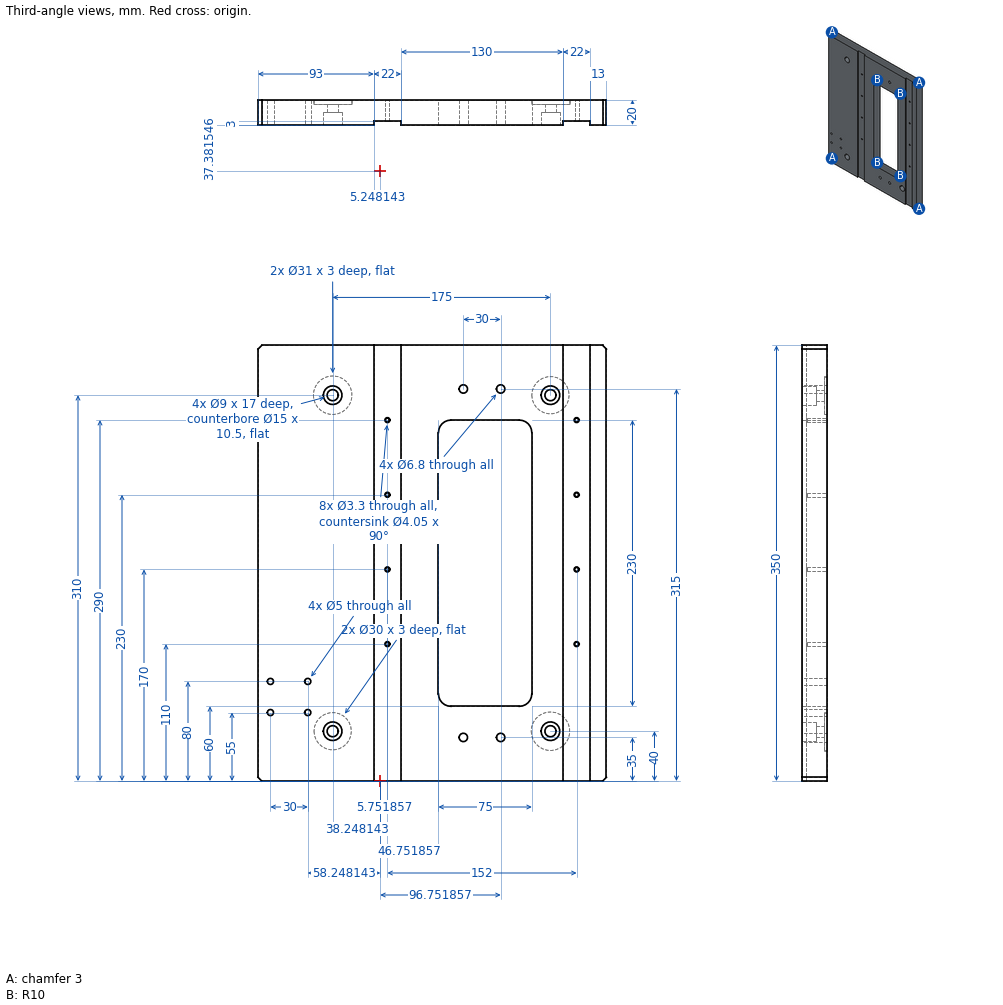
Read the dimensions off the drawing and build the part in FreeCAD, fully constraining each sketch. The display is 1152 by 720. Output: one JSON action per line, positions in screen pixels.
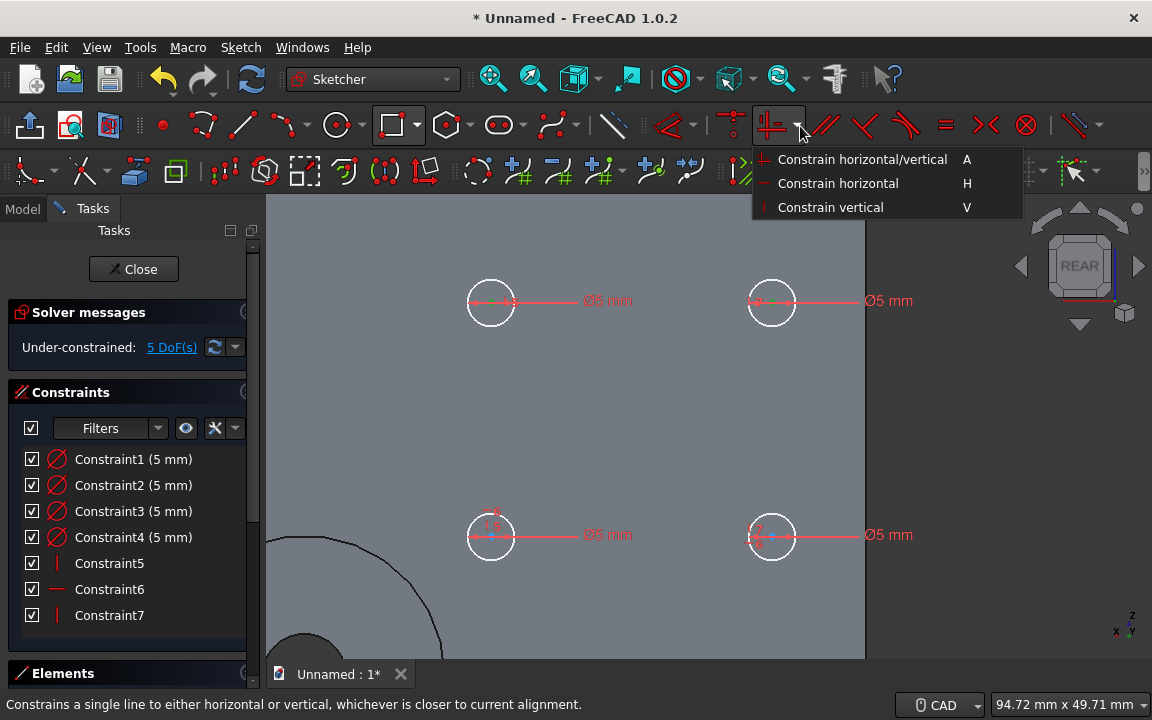
{"action": "left_click", "coordinate": [888, 183]}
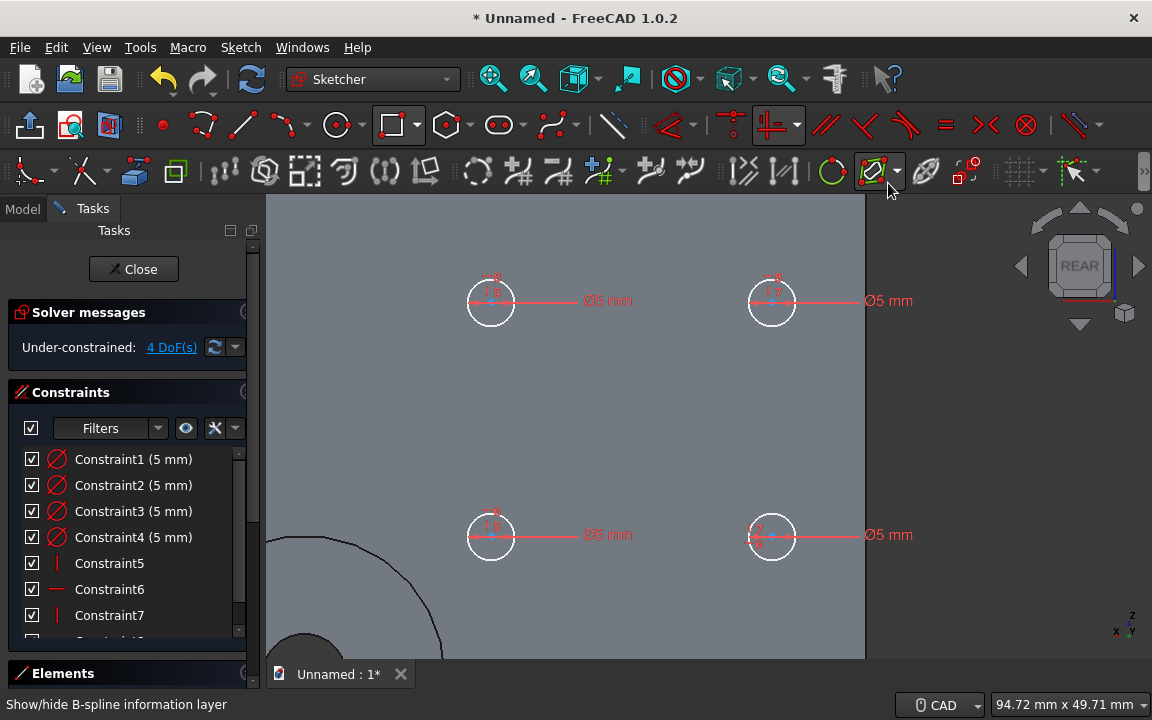
{"action": "left_click", "coordinate": [668, 126]}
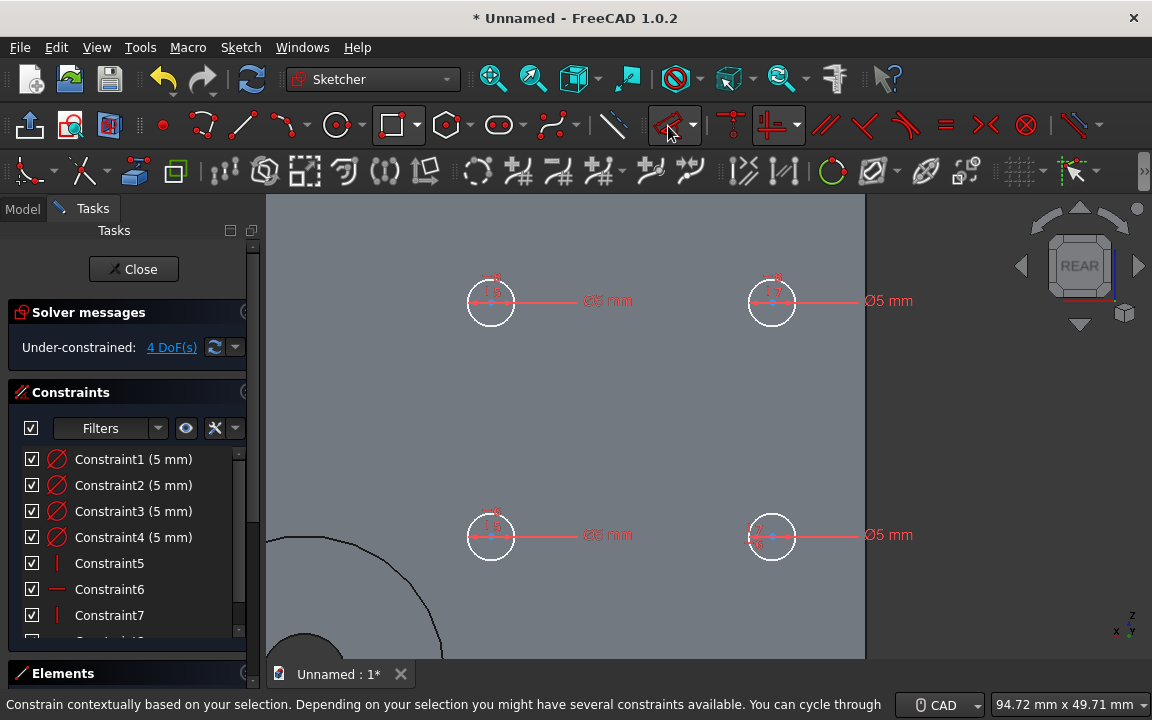
{"action": "left_click", "coordinate": [491, 303]}
{"action": "left_click", "coordinate": [525, 467]}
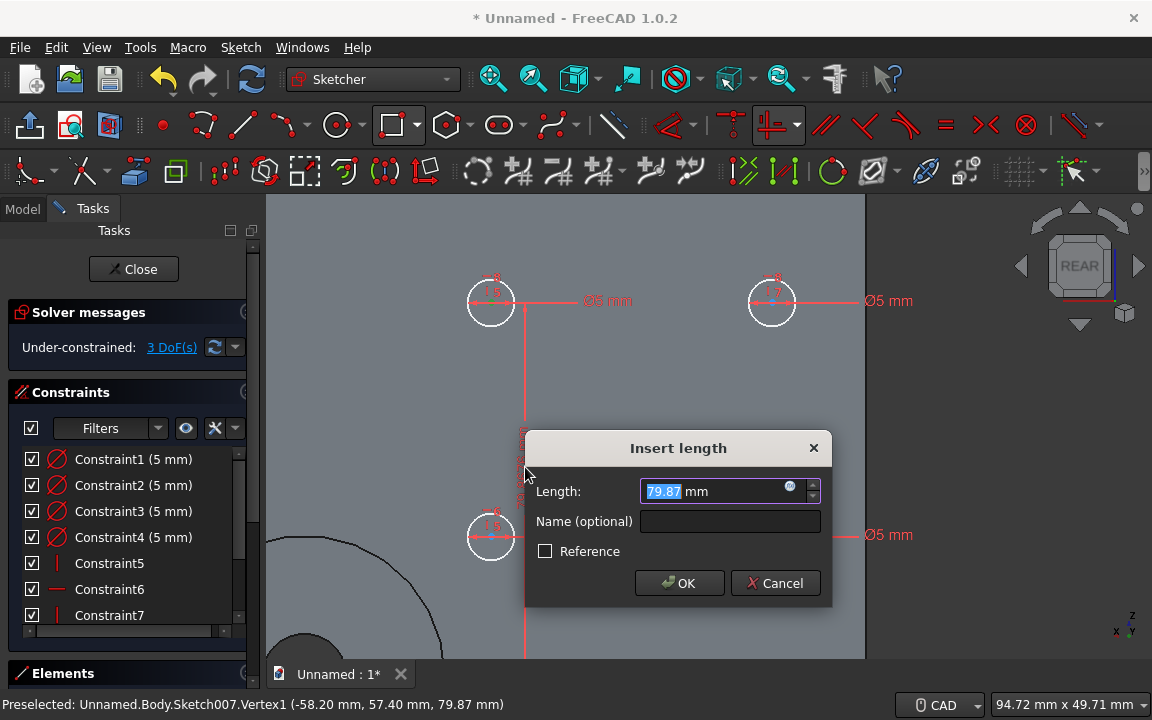
{"action": "type", "text": "80"}
{"action": "key", "text": "Return"}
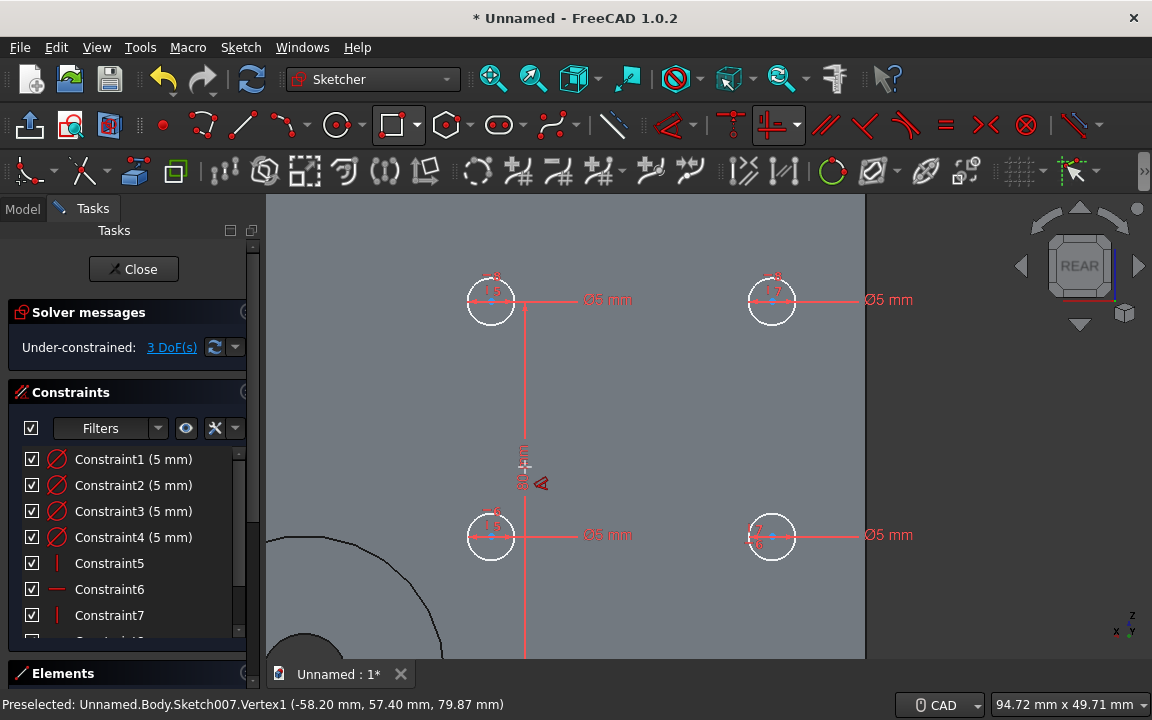
{"action": "left_click", "coordinate": [491, 537]}
{"action": "left_click", "coordinate": [525, 584]}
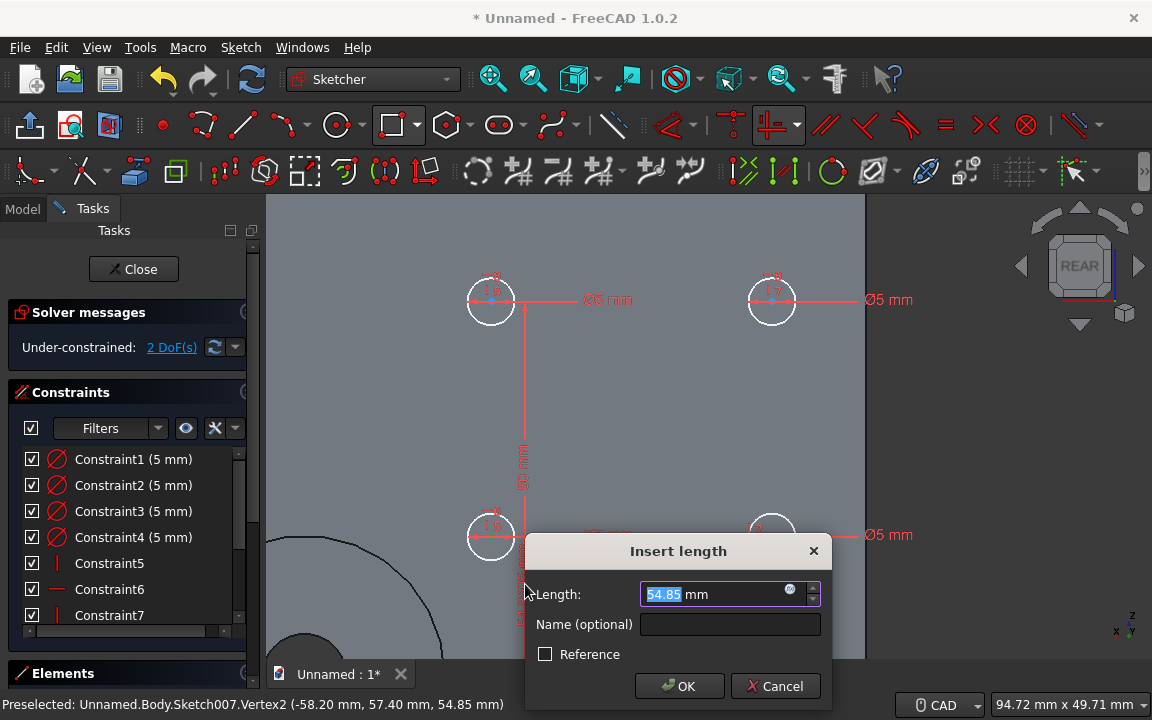
{"action": "type", "text": "55"}
{"action": "key", "text": "Return"}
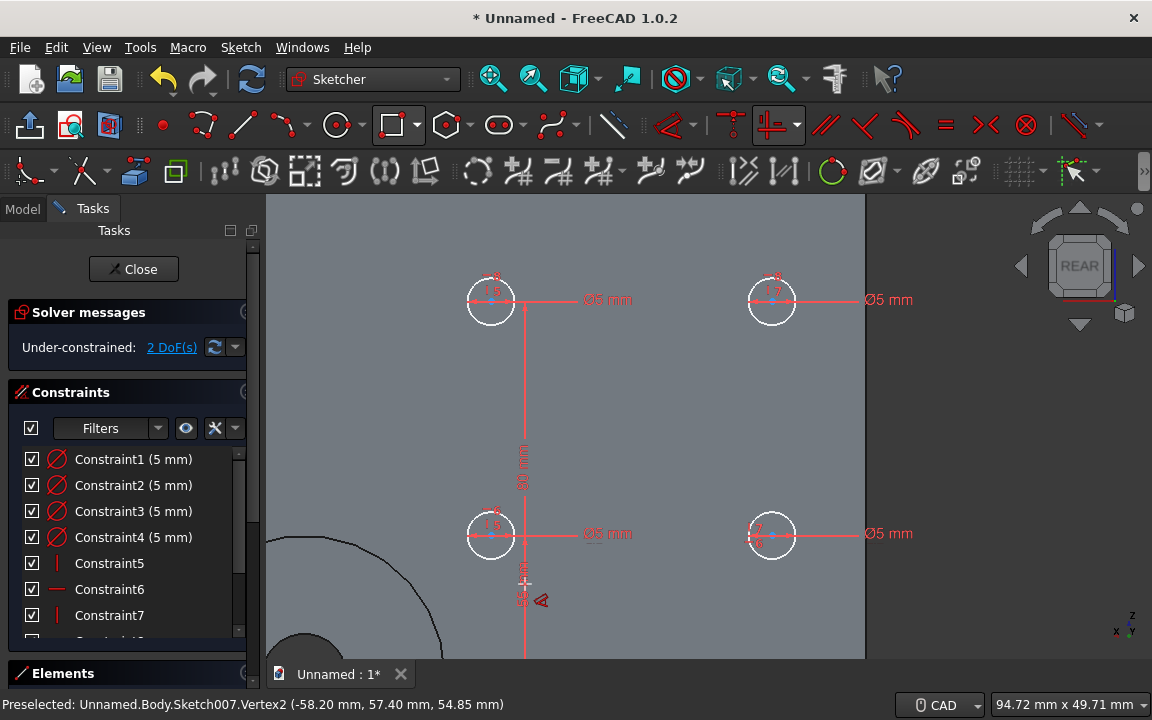
{"action": "left_click", "coordinate": [491, 536]}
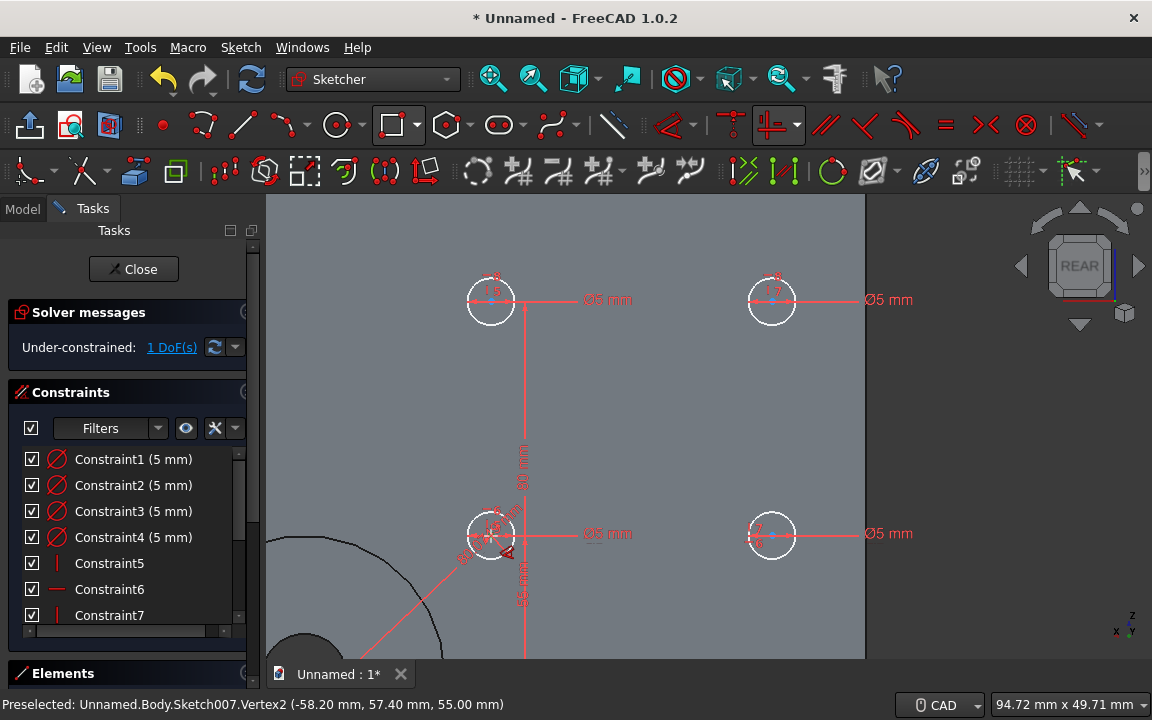
{"action": "left_click", "coordinate": [772, 536]}
{"action": "left_click", "coordinate": [631, 570]}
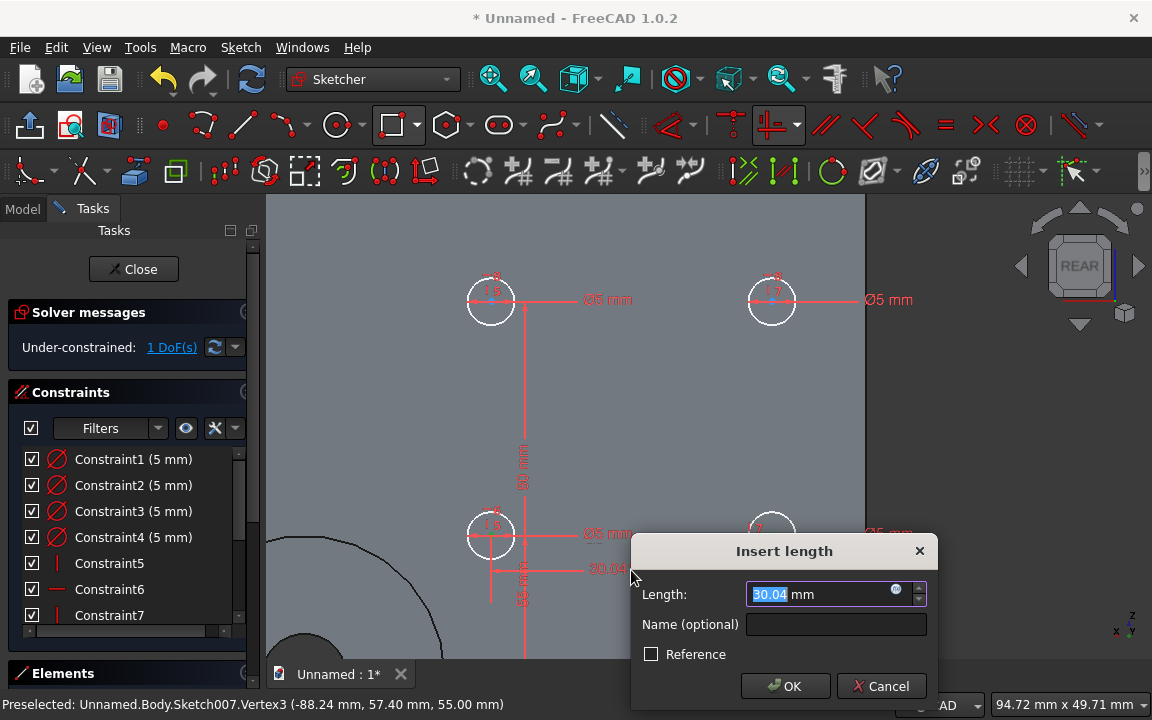
{"action": "type", "text": "30"}
{"action": "key", "text": "Return"}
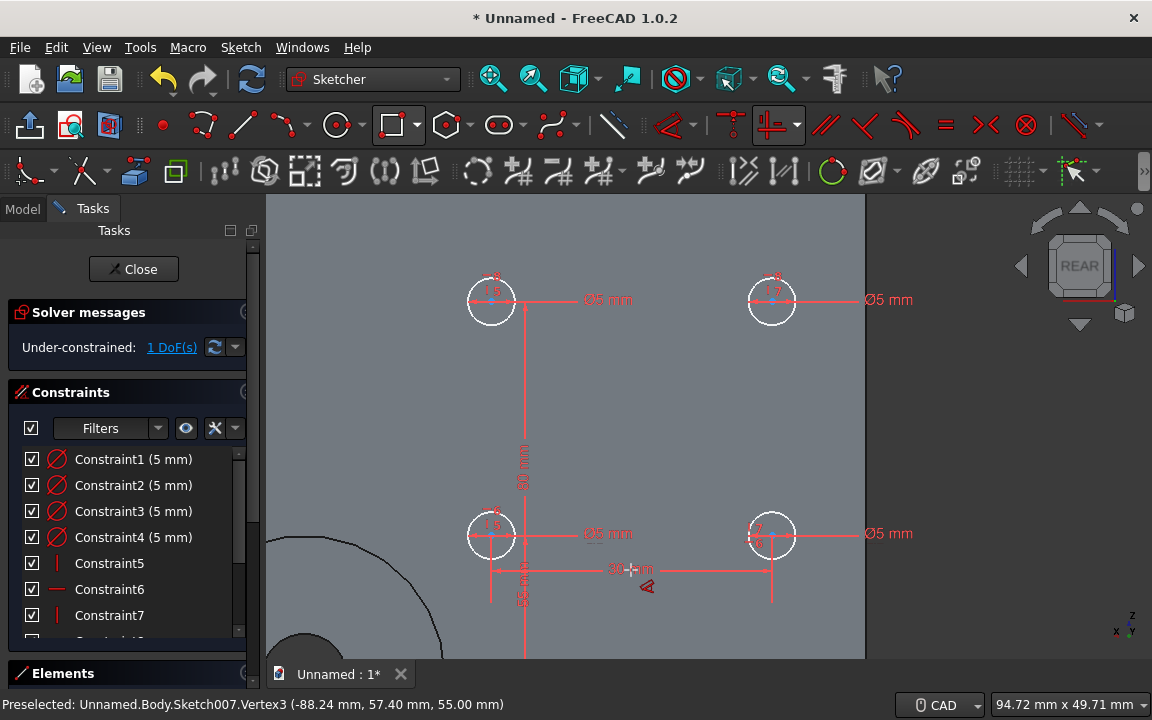
{"action": "left_click", "coordinate": [491, 302]}
{"action": "left_click", "coordinate": [393, 268]}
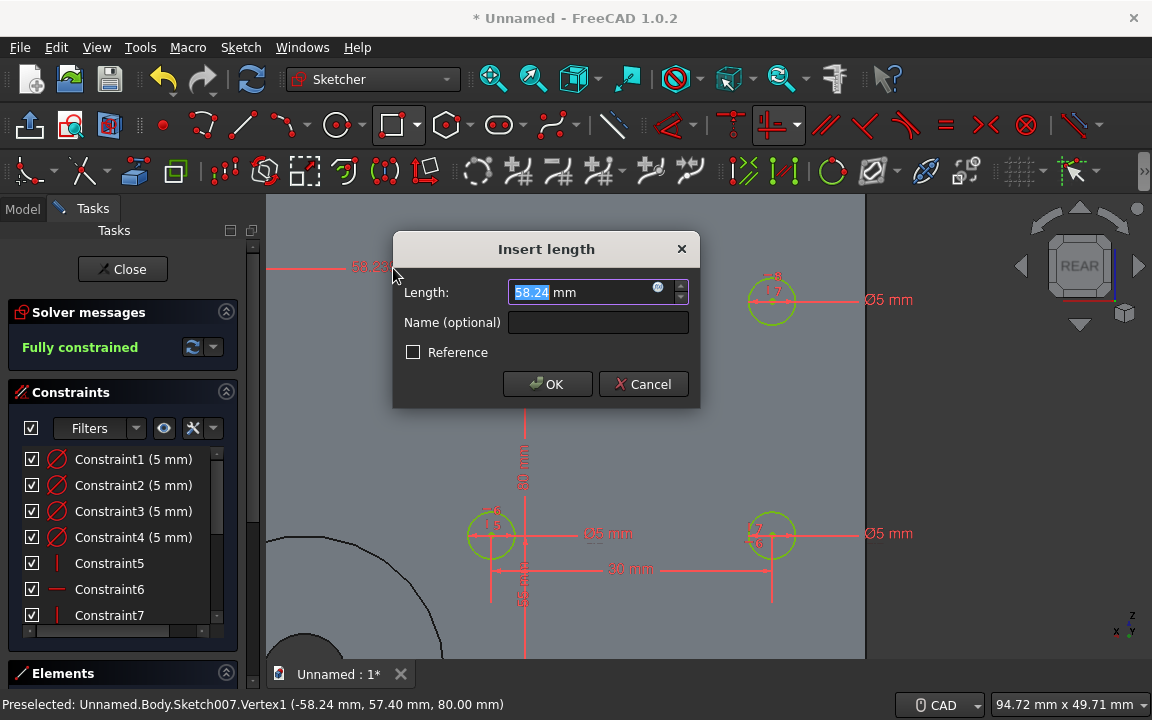
{"action": "type", "text": "58.248143"}
{"action": "key", "text": "Return"}
{"action": "key", "text": "Escape"}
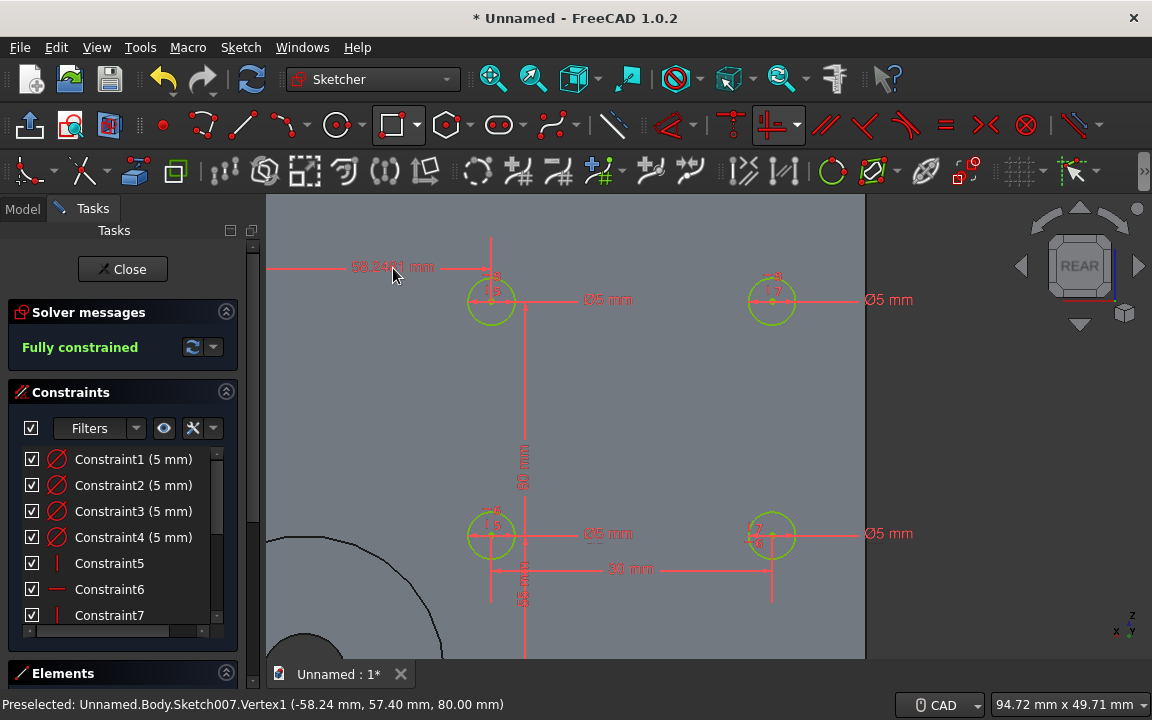
{"action": "left_click", "coordinate": [123, 269]}